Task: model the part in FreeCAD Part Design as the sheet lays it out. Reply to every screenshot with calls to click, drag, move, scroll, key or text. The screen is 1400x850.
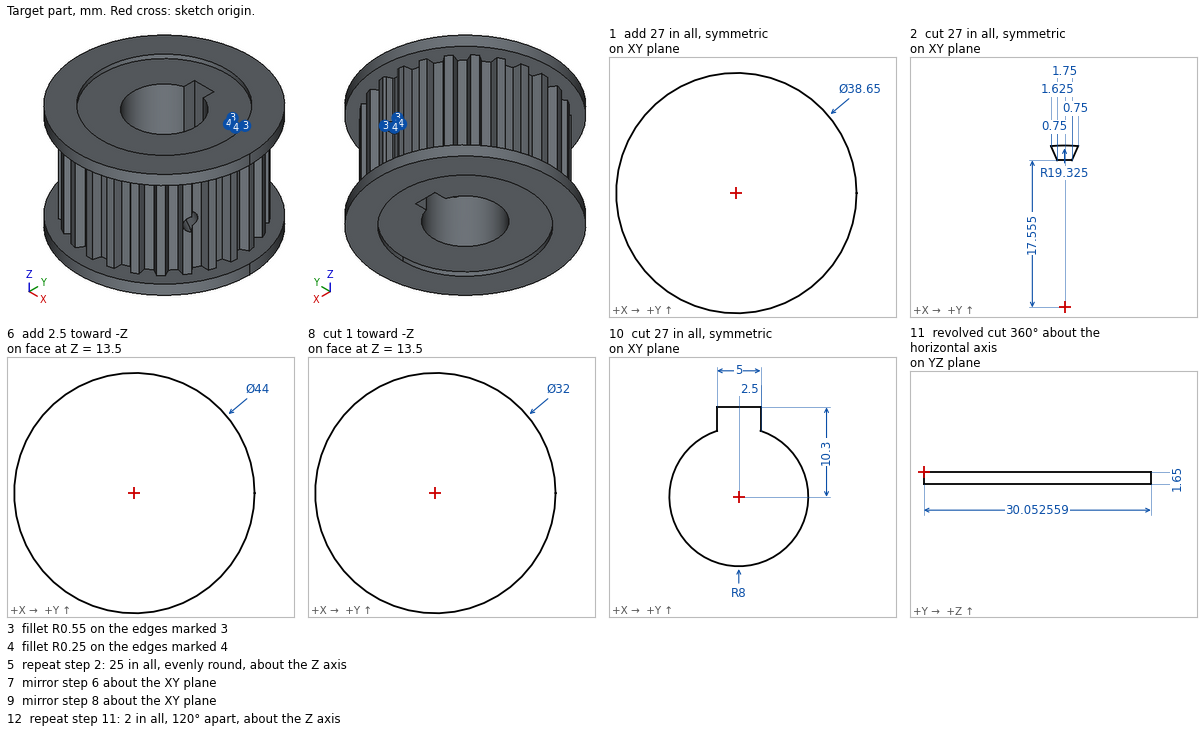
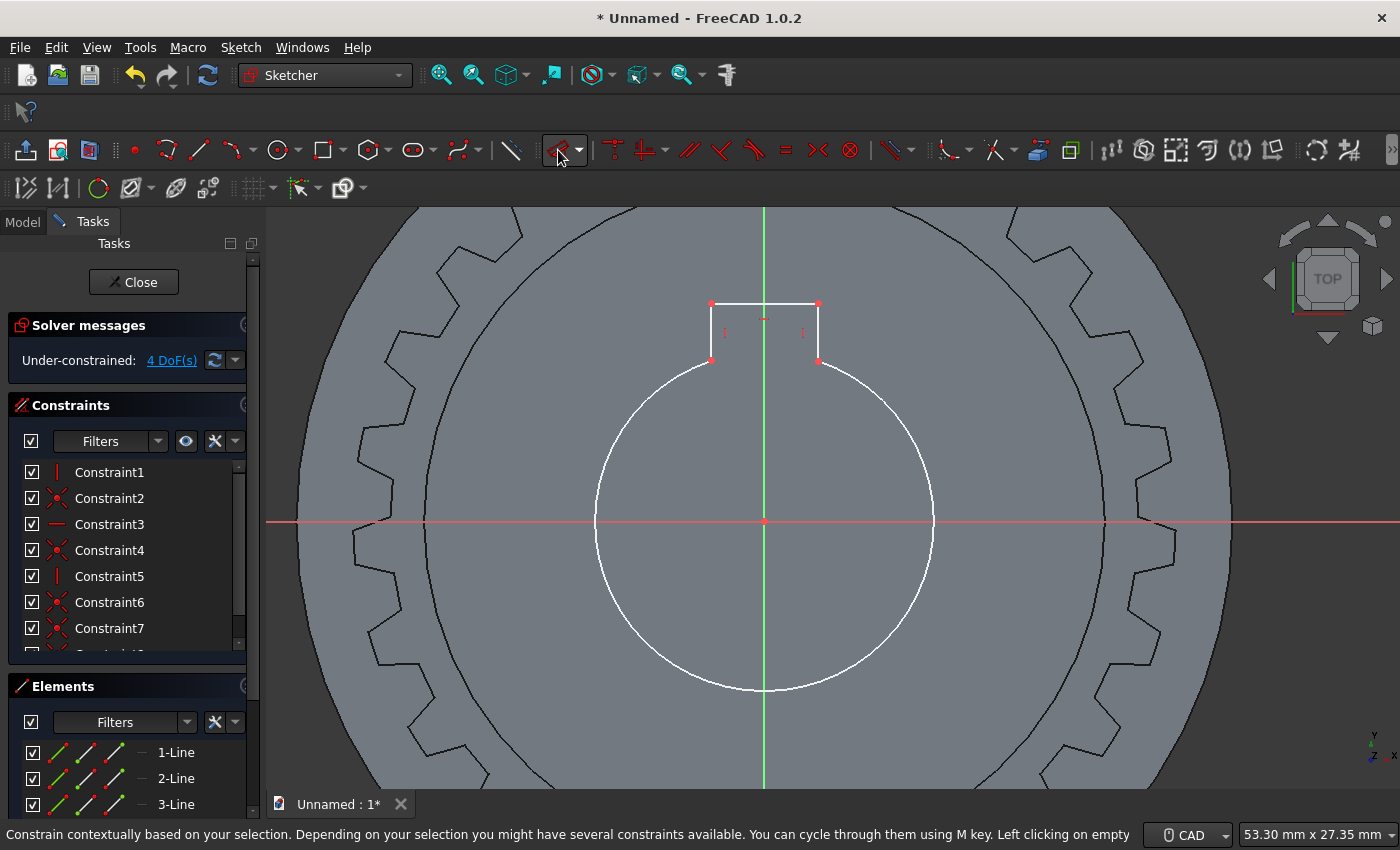
click(611, 594)
click(582, 608)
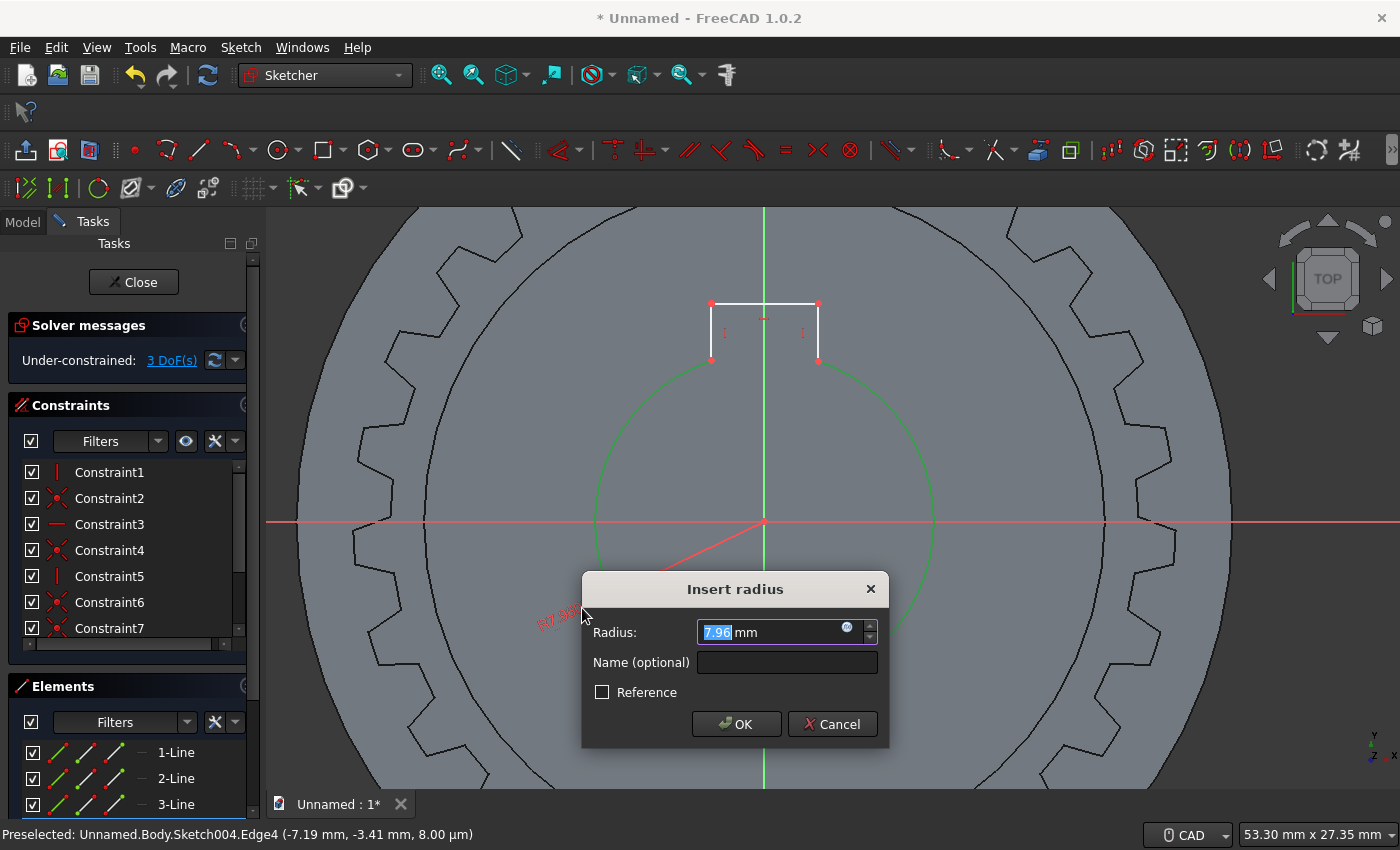
text(8)
key(Return)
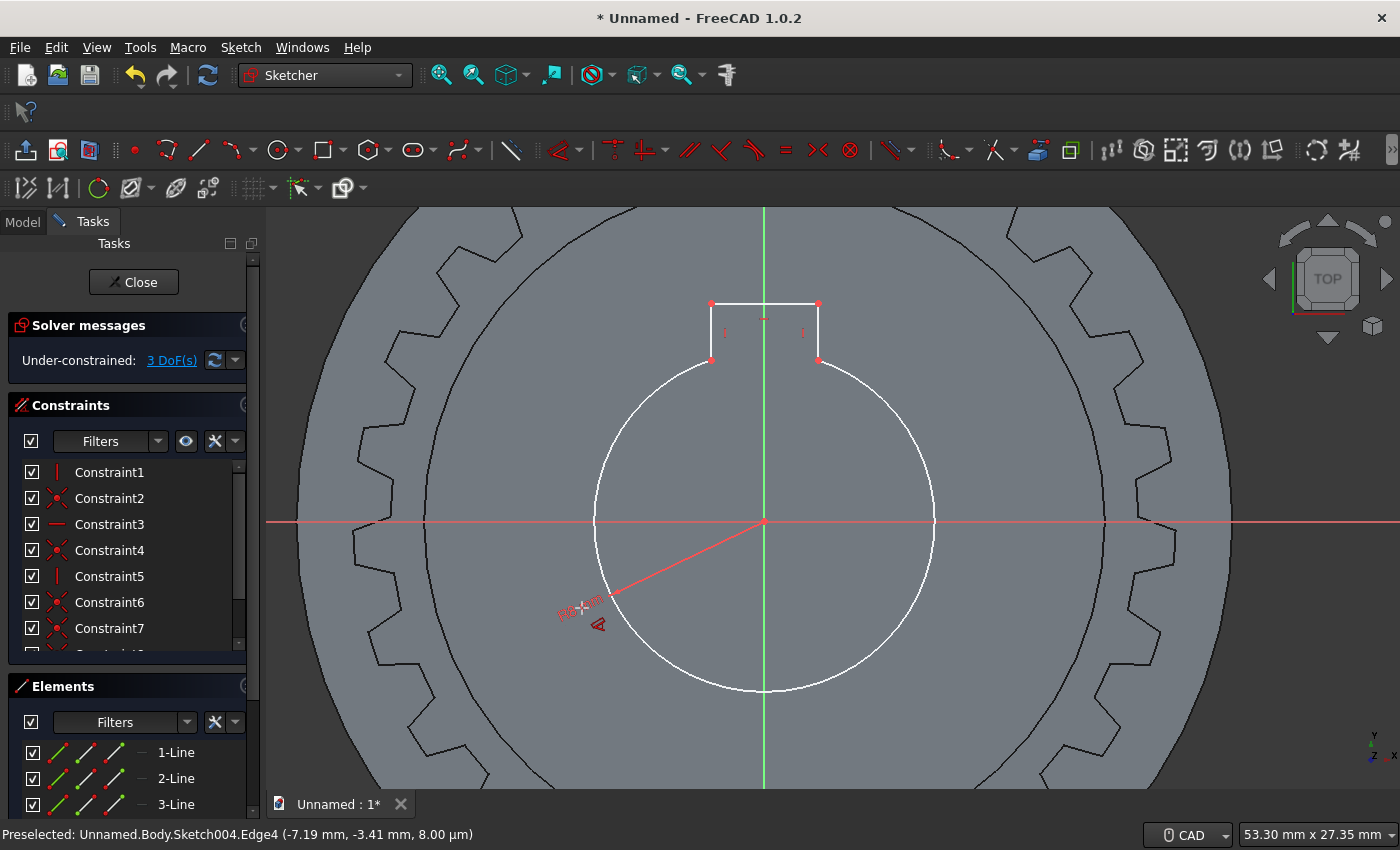
click(786, 304)
click(740, 270)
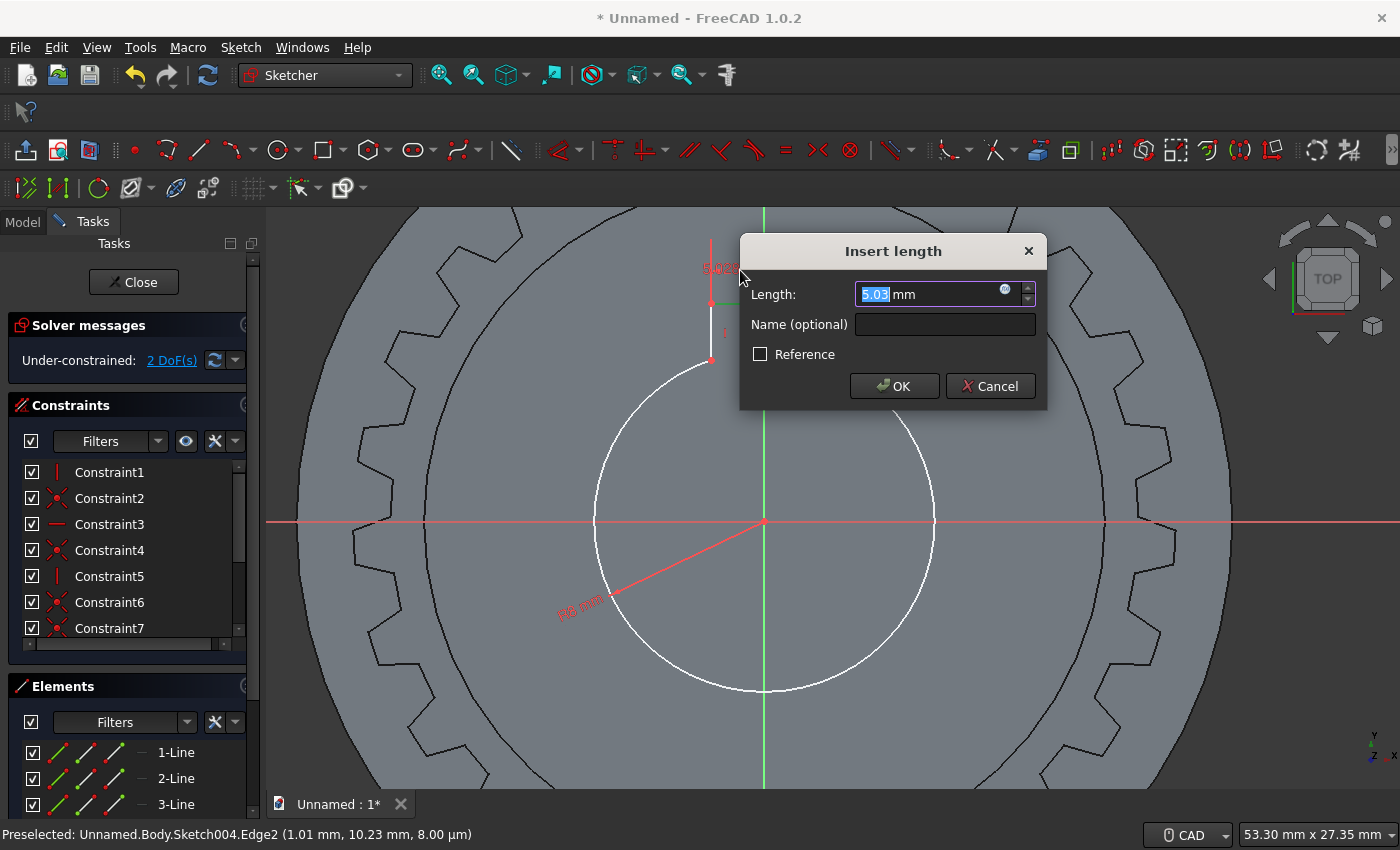
text(5)
key(Return)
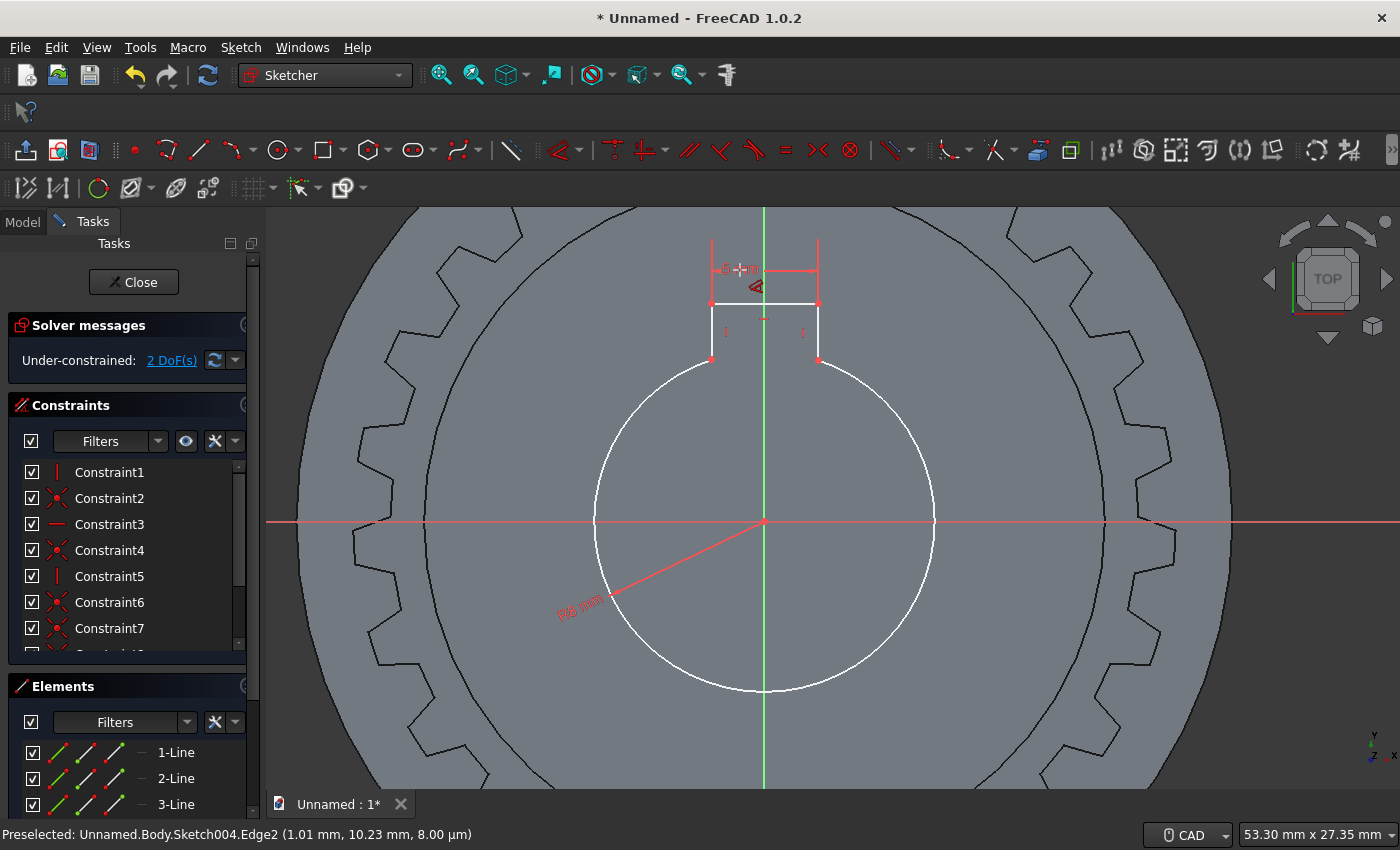
click(818, 360)
click(791, 326)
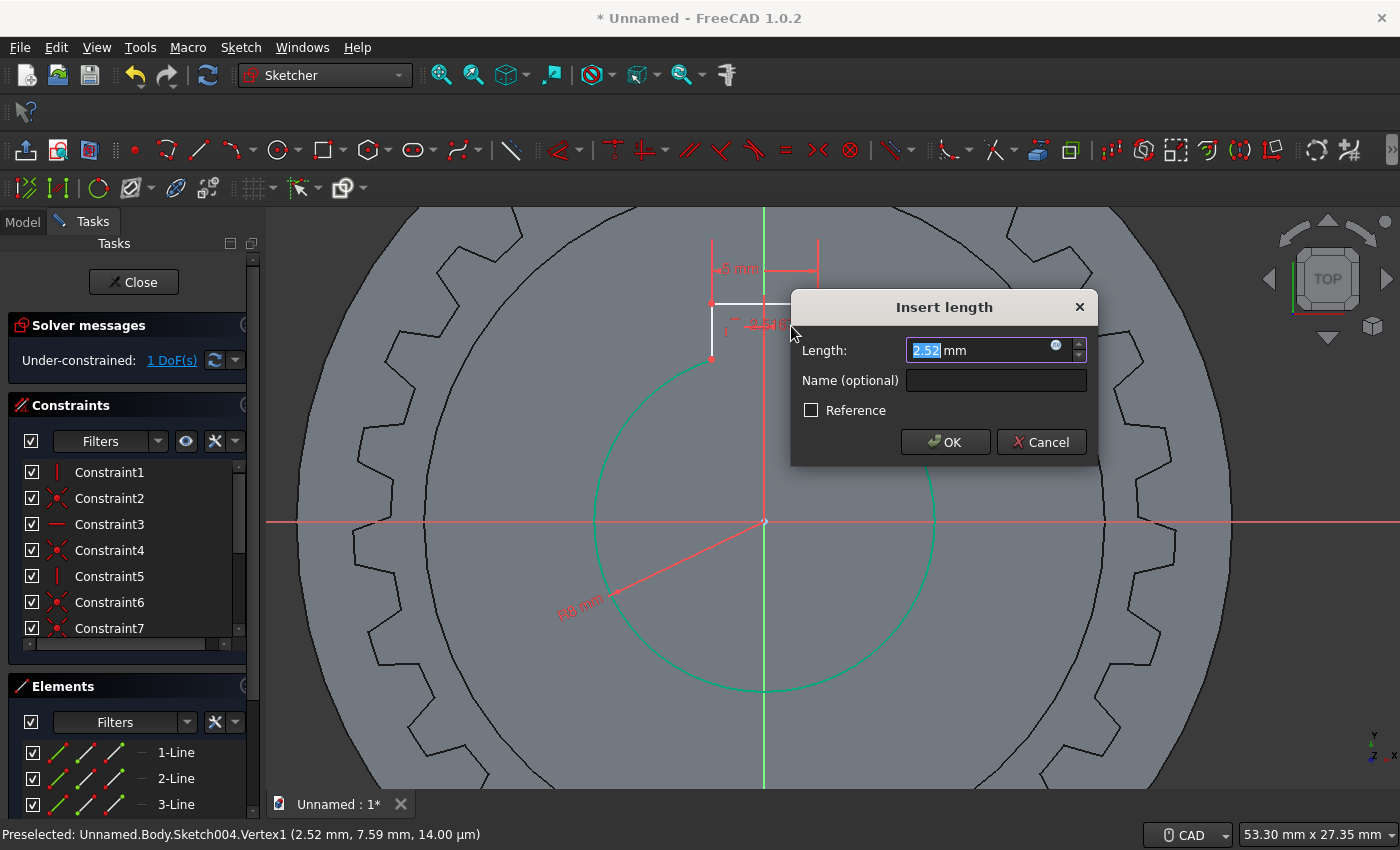
text(2.5)
key(Return)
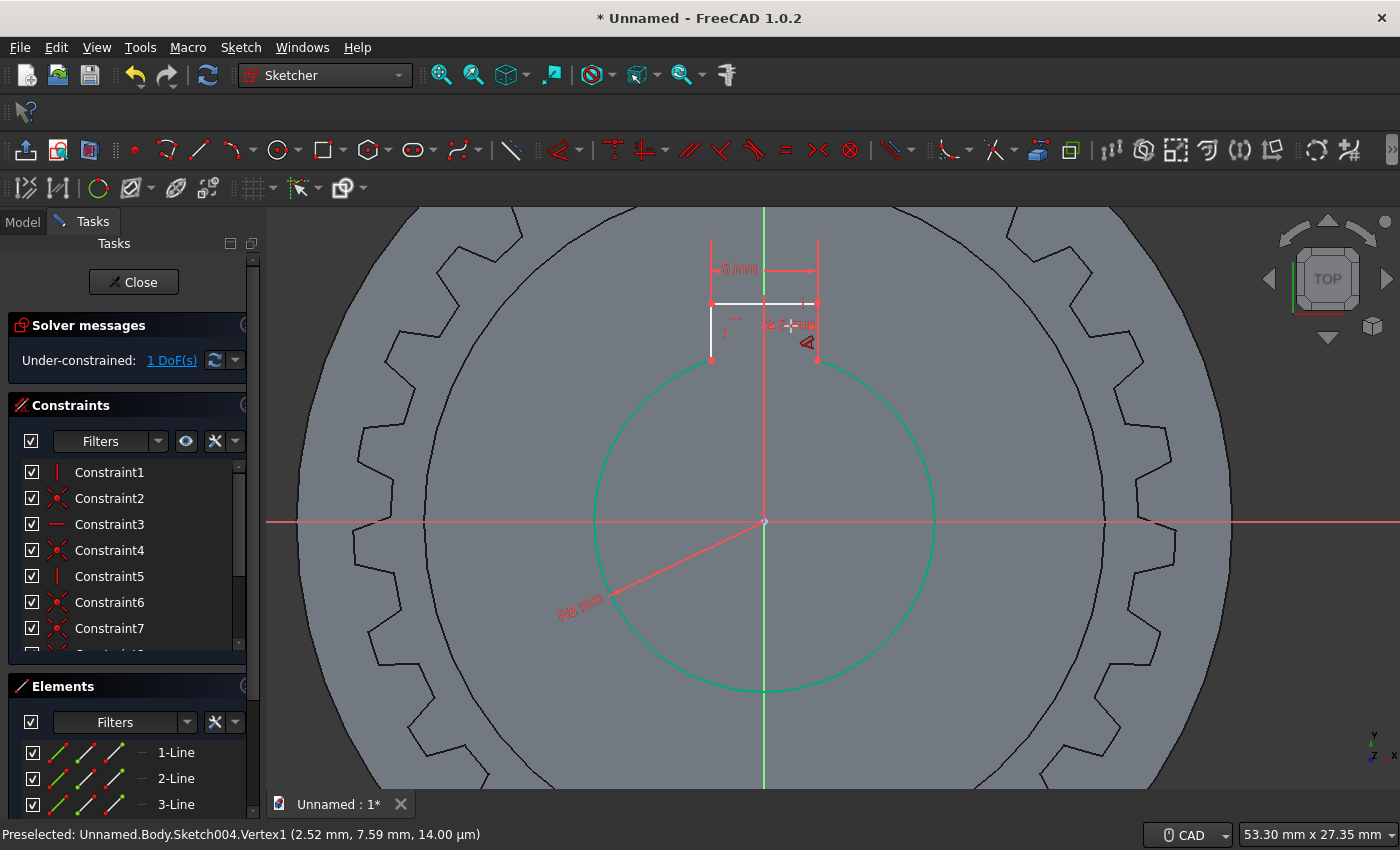
click(818, 304)
click(852, 413)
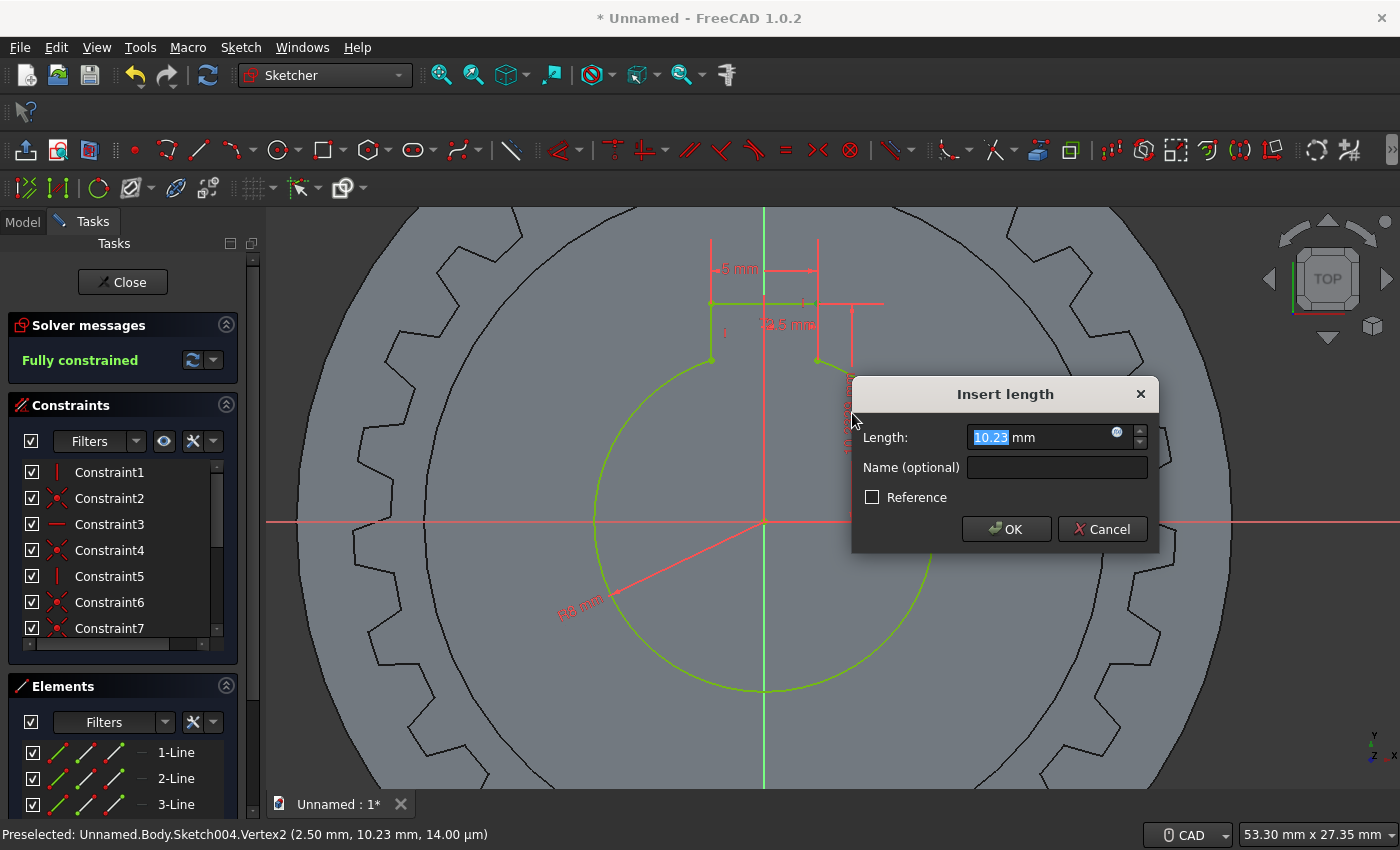
text(10.3)
key(Return)
key(Escape)